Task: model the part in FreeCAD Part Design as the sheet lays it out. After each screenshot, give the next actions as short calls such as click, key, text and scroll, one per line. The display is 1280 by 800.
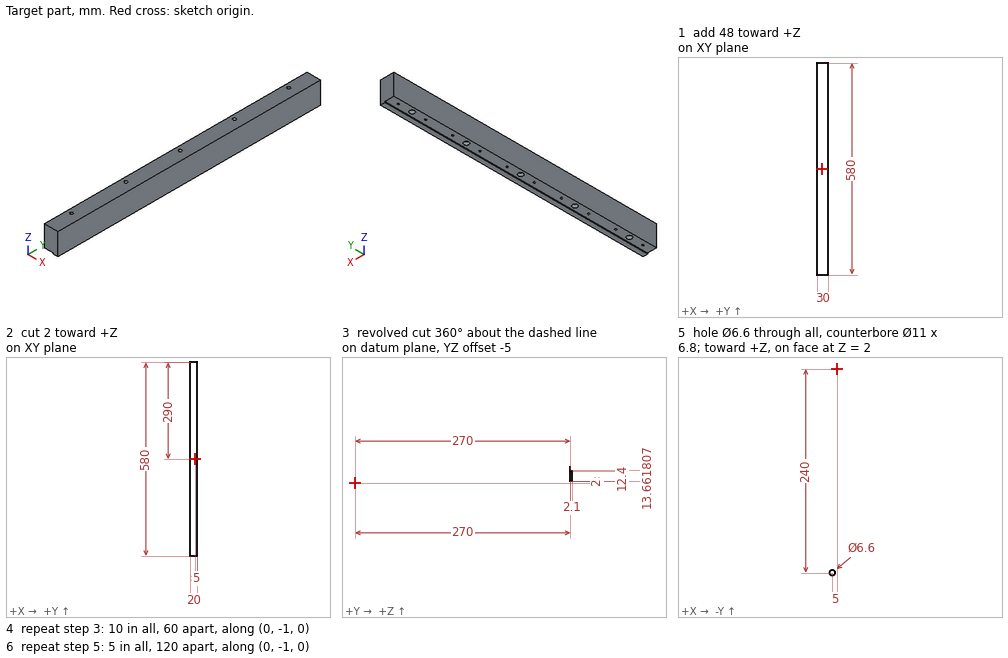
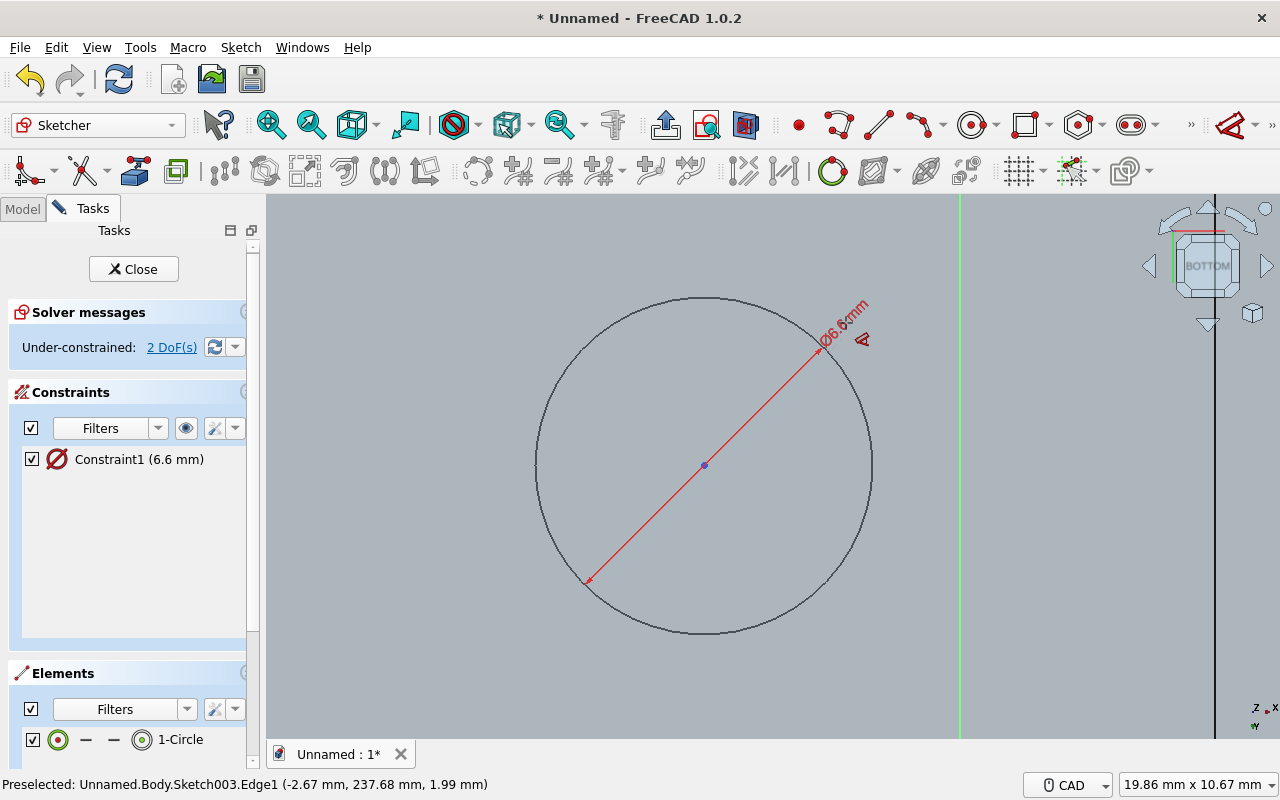
click(704, 466)
click(832, 500)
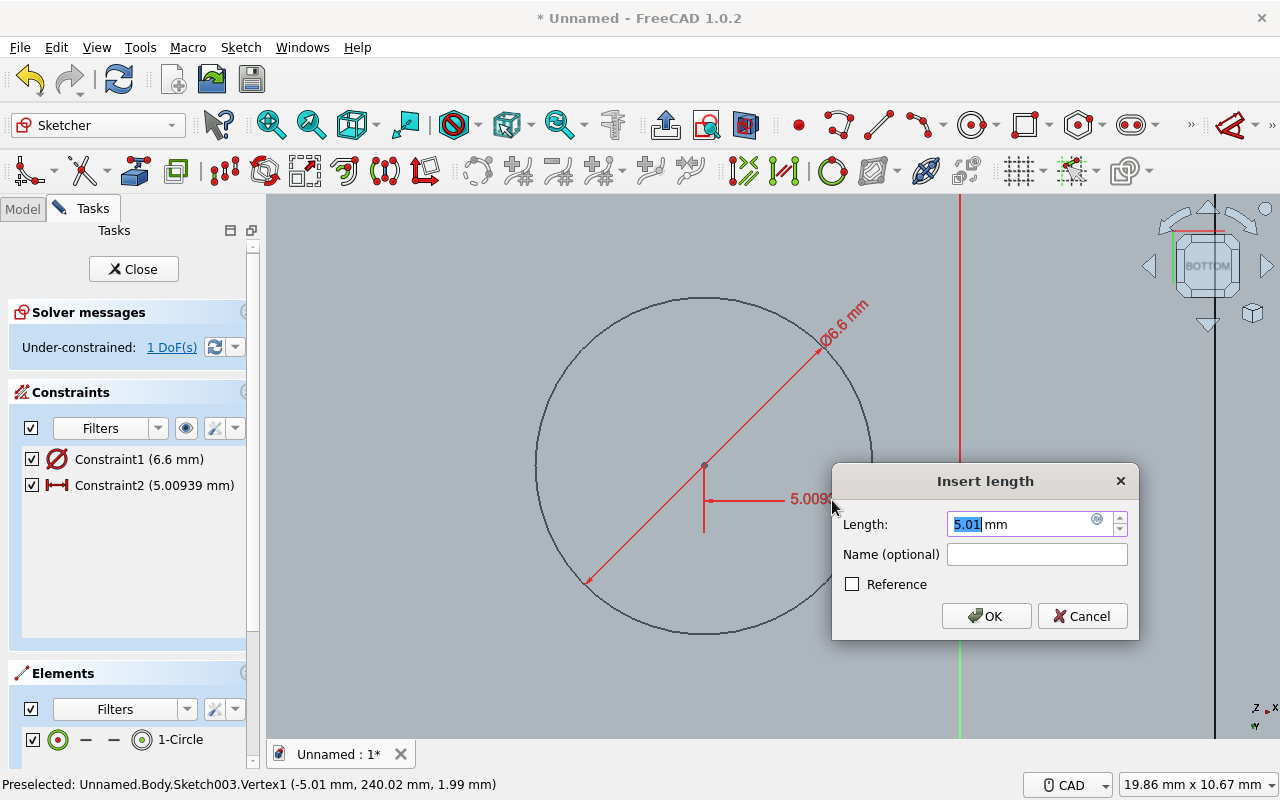
text(5)
key(Return)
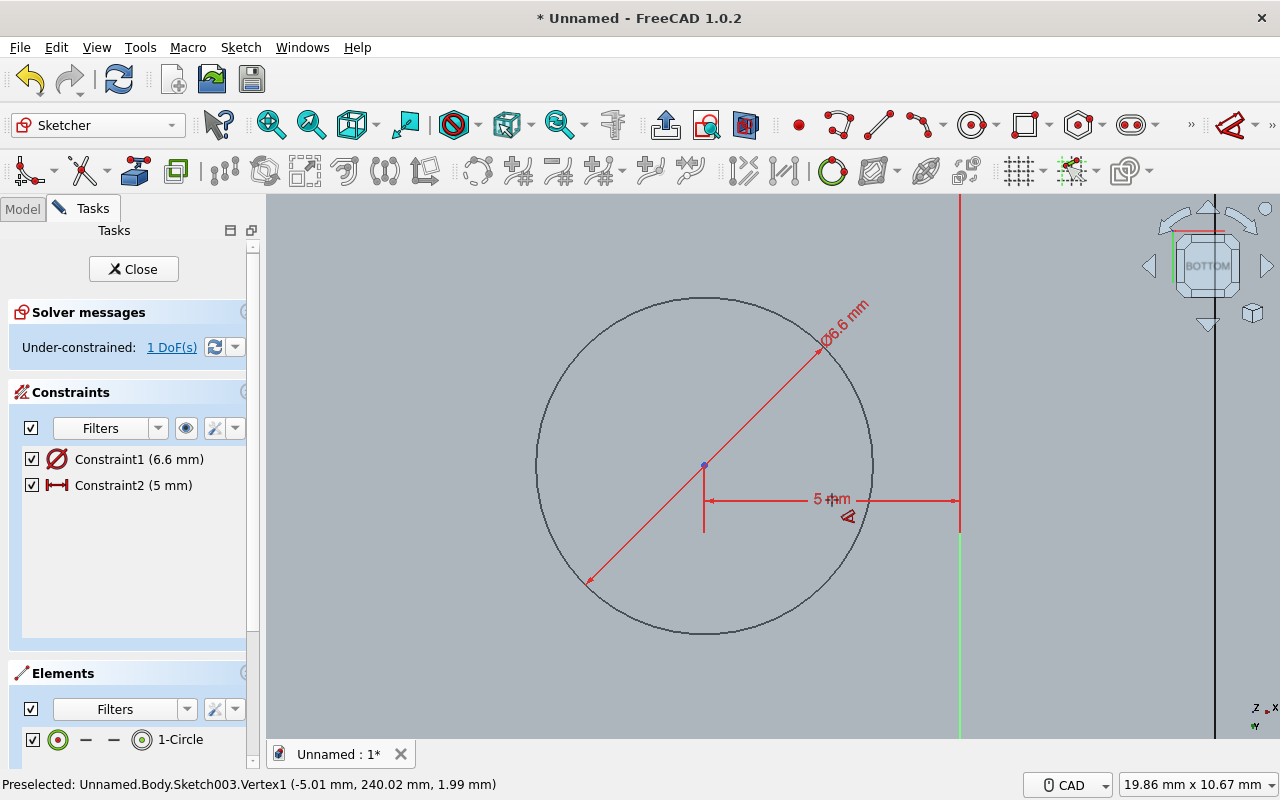
click(704, 466)
click(994, 344)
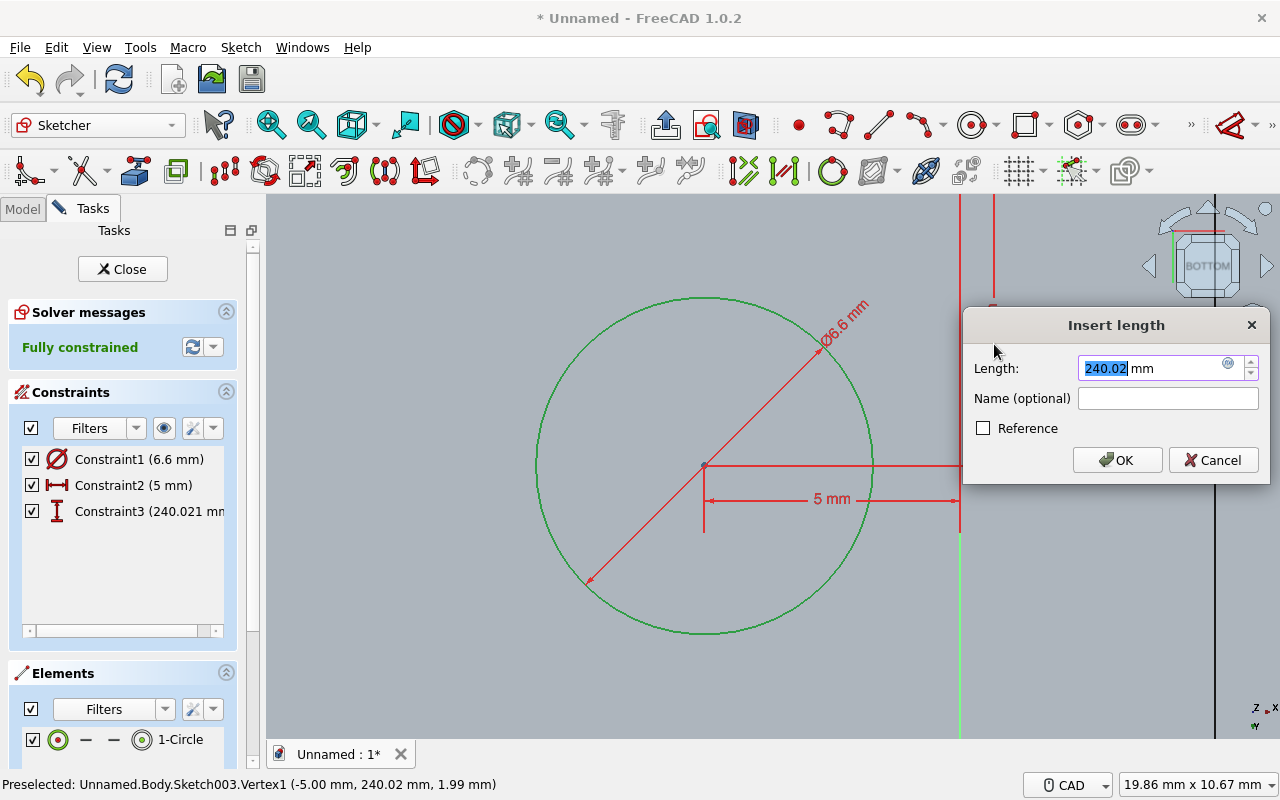
text(240)
key(Return)
key(Escape)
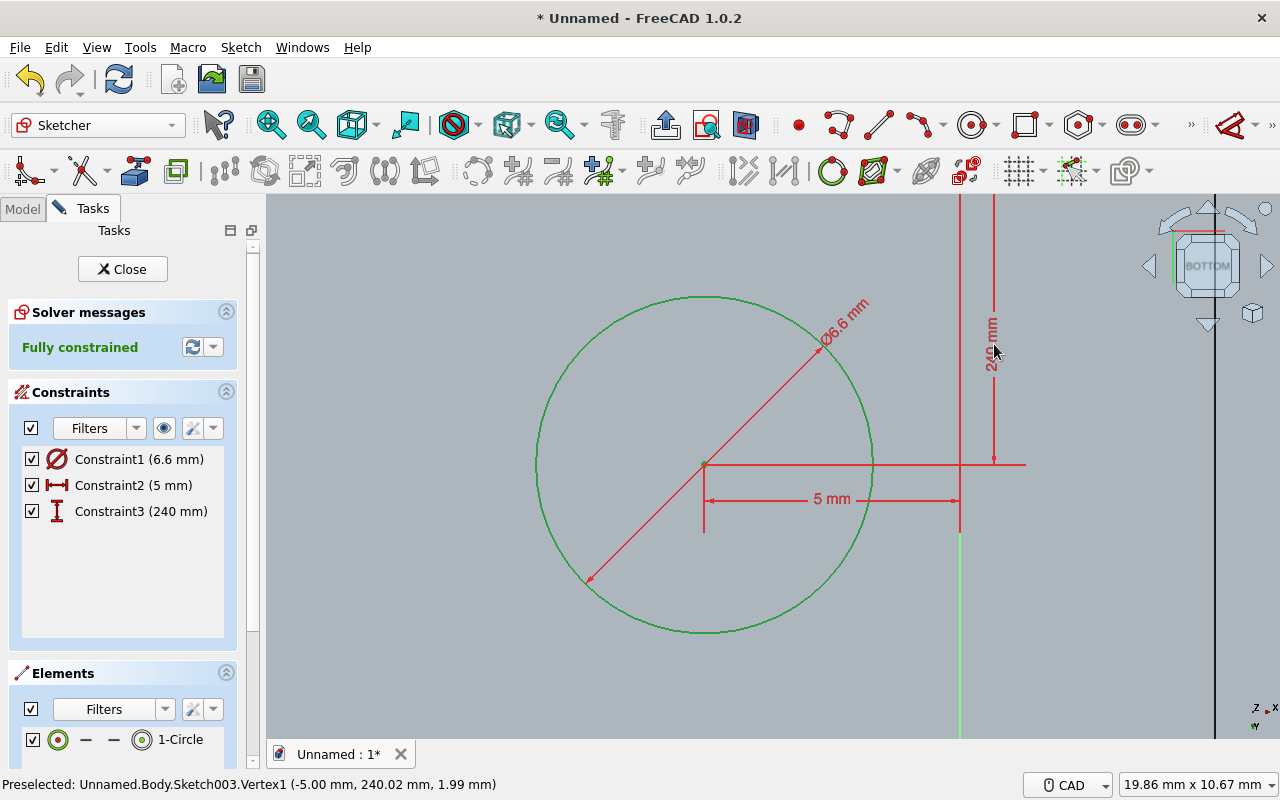
click(123, 269)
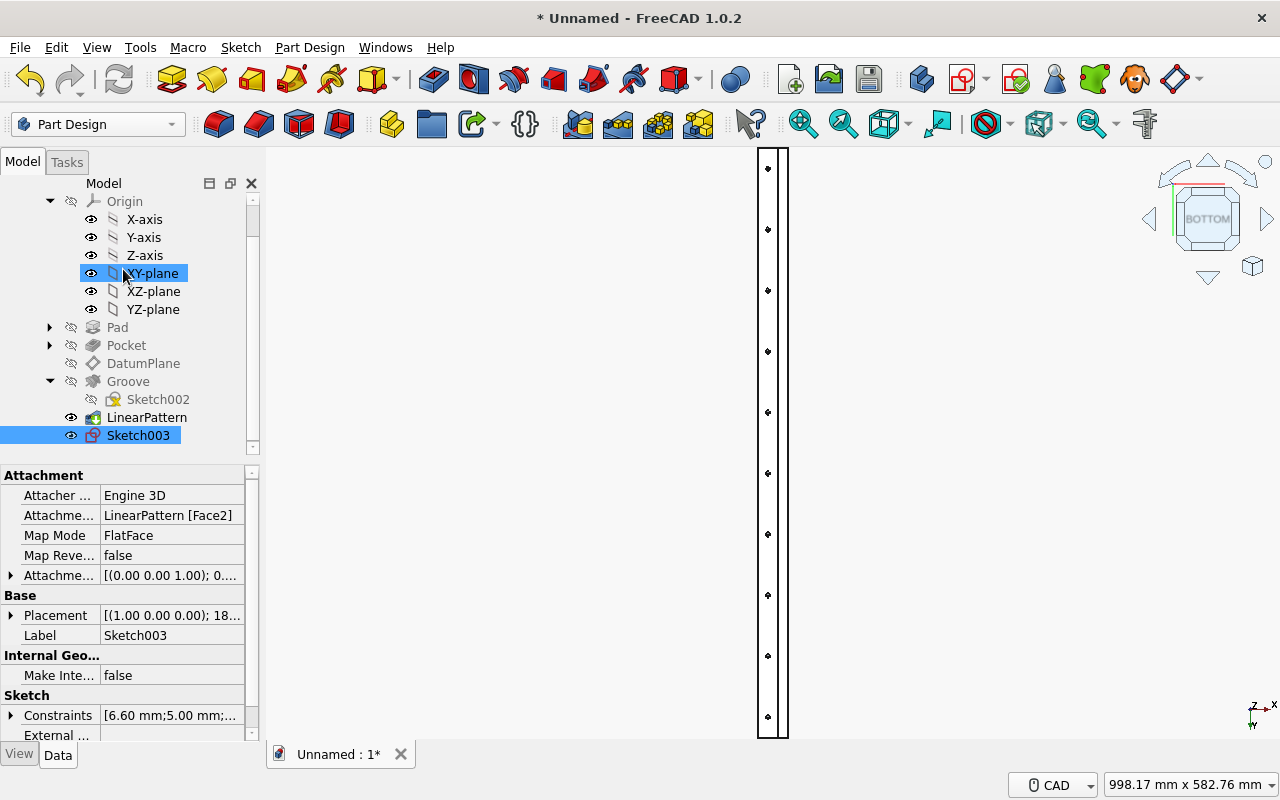
click(474, 80)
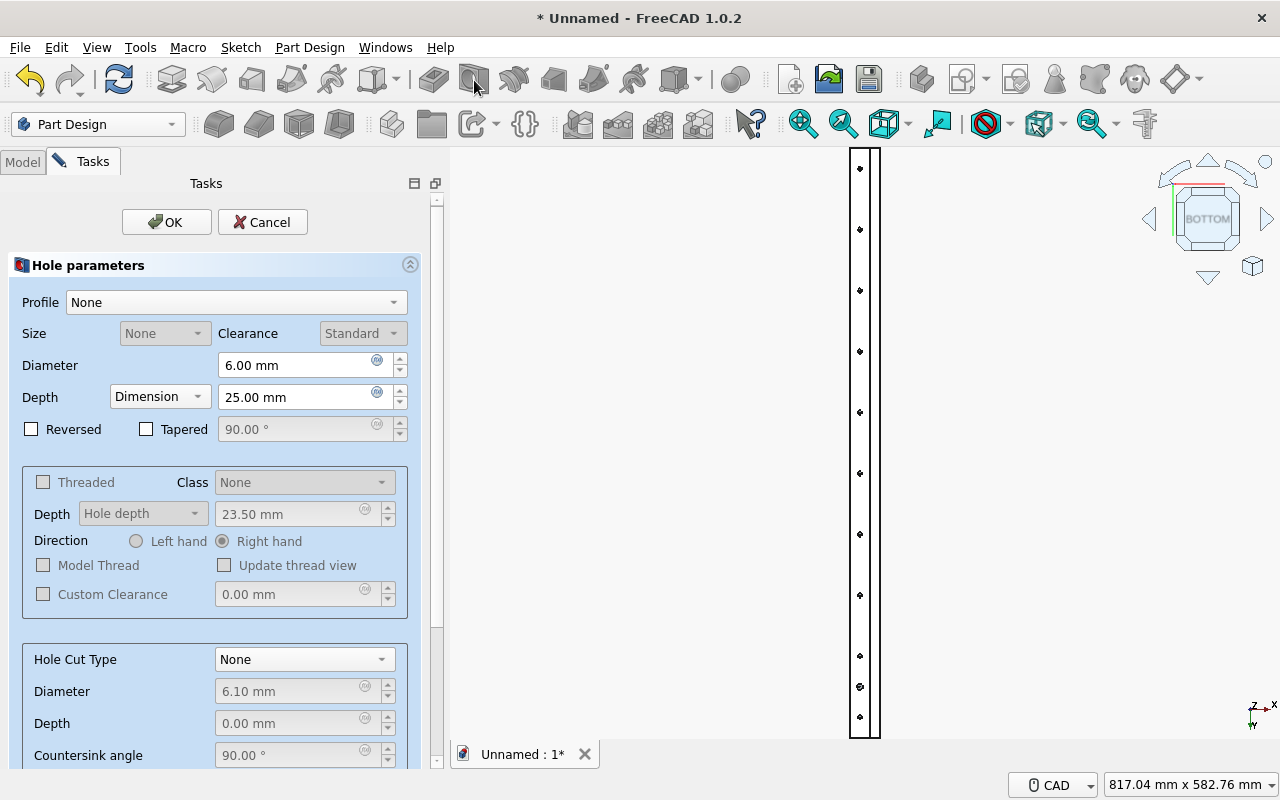
triple_click(305, 365)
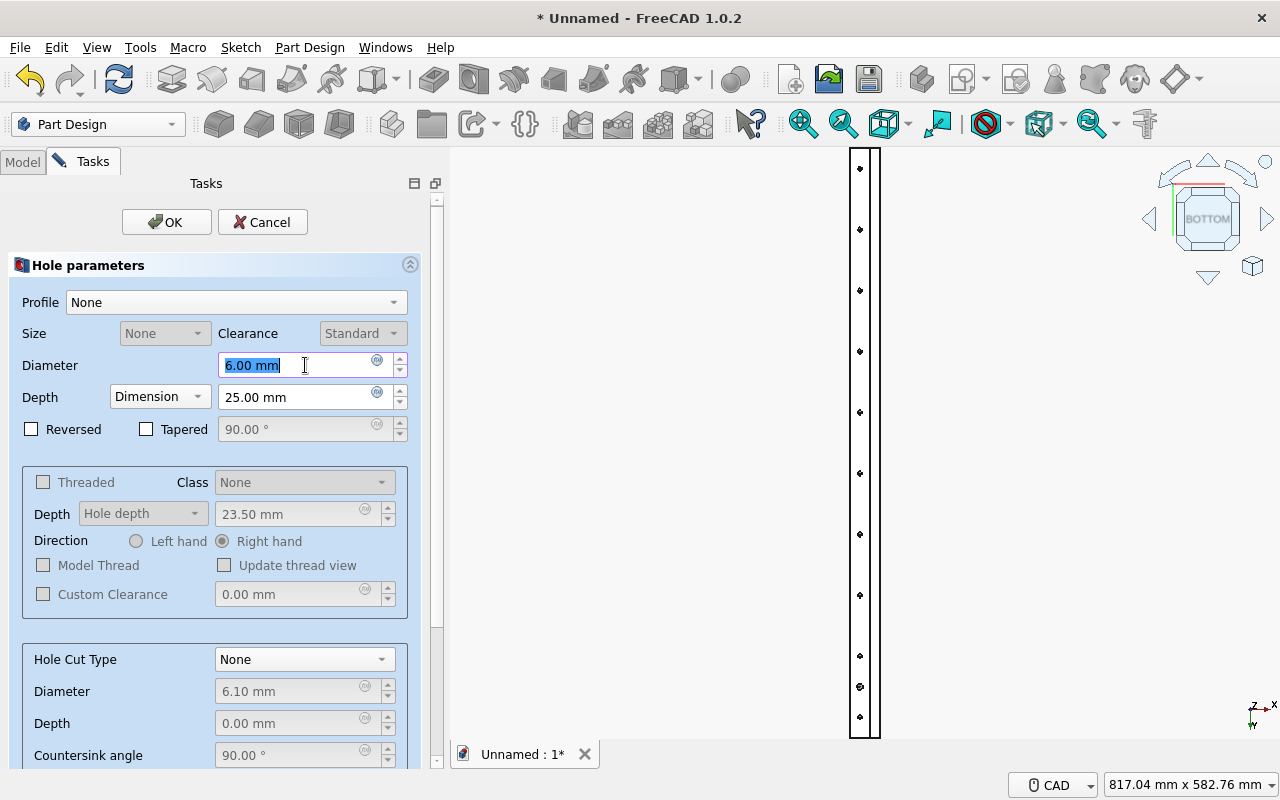
text(6.6)
key(Tab)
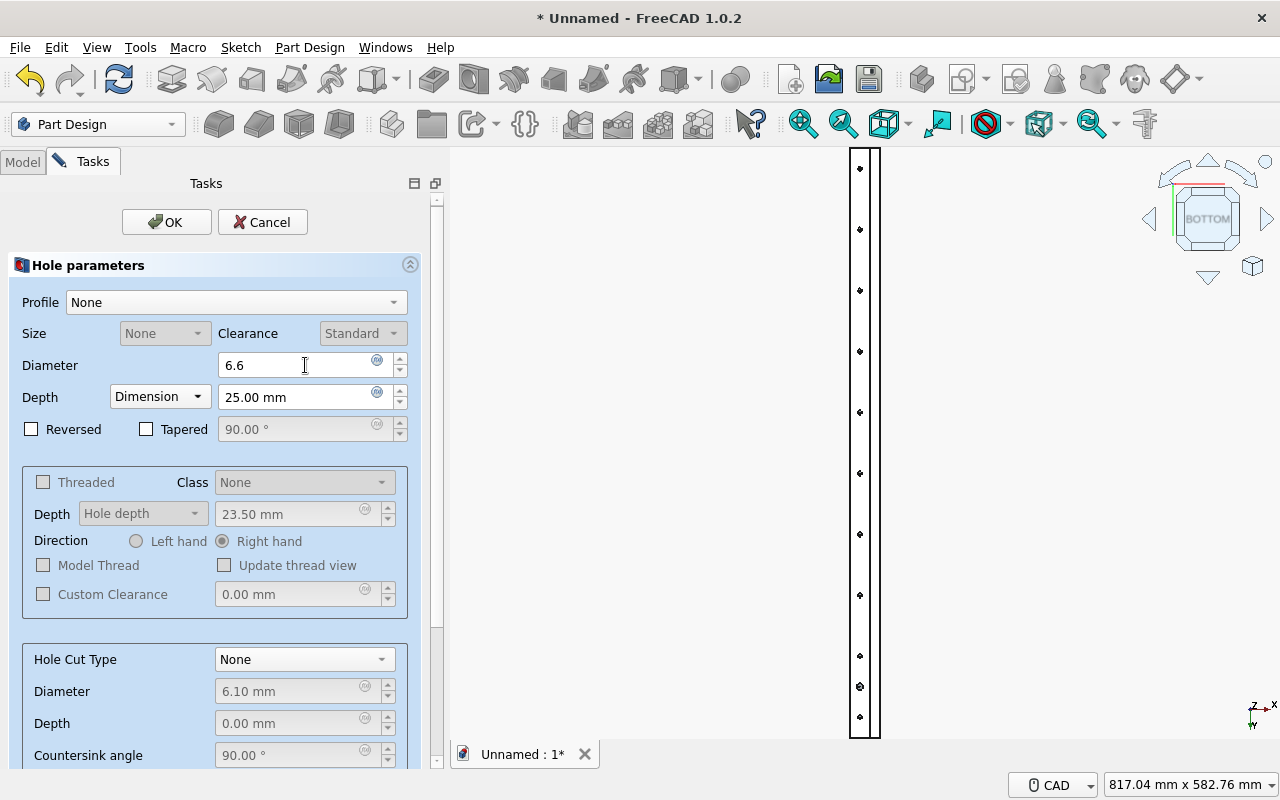
click(161, 396)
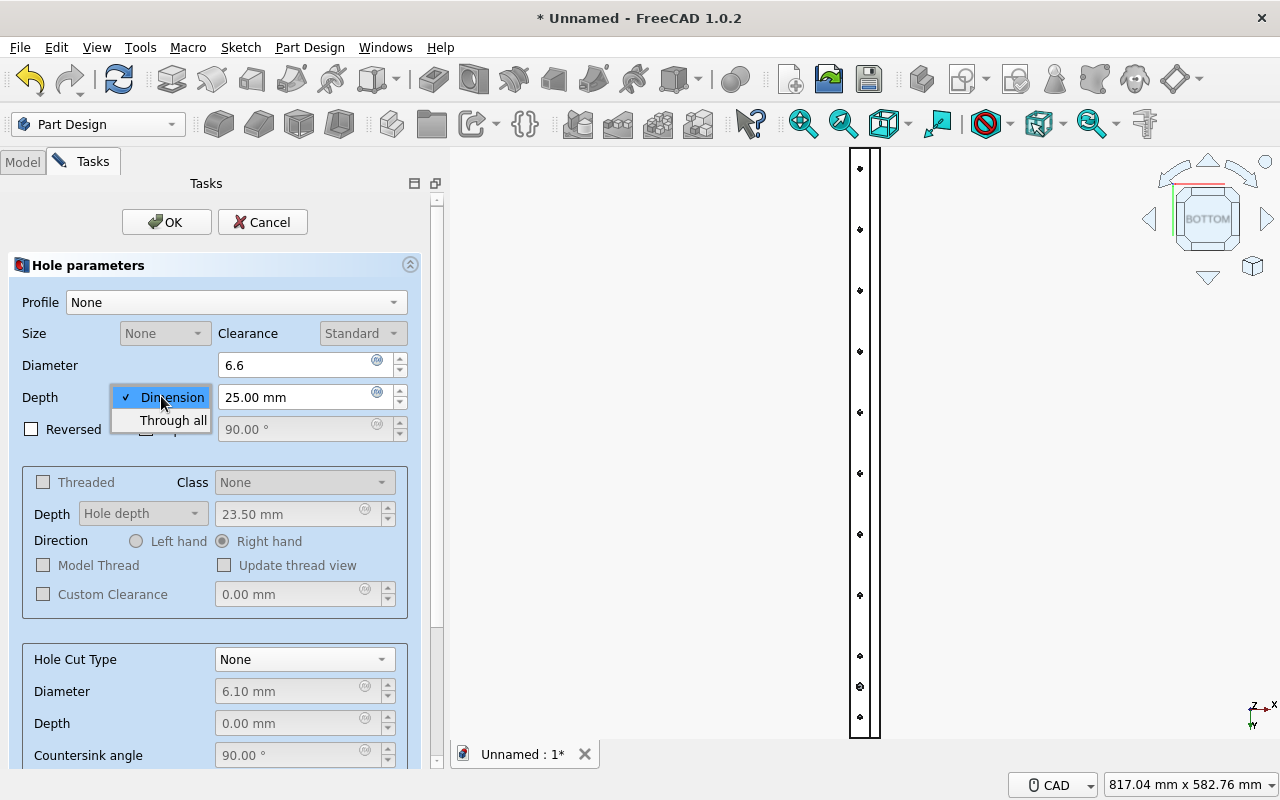
click(160, 420)